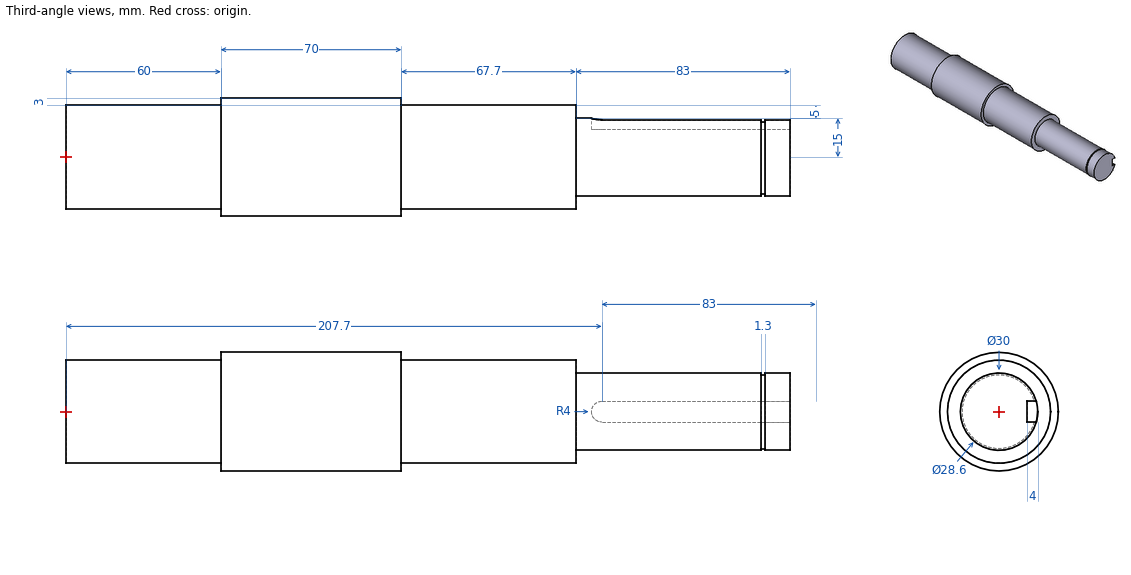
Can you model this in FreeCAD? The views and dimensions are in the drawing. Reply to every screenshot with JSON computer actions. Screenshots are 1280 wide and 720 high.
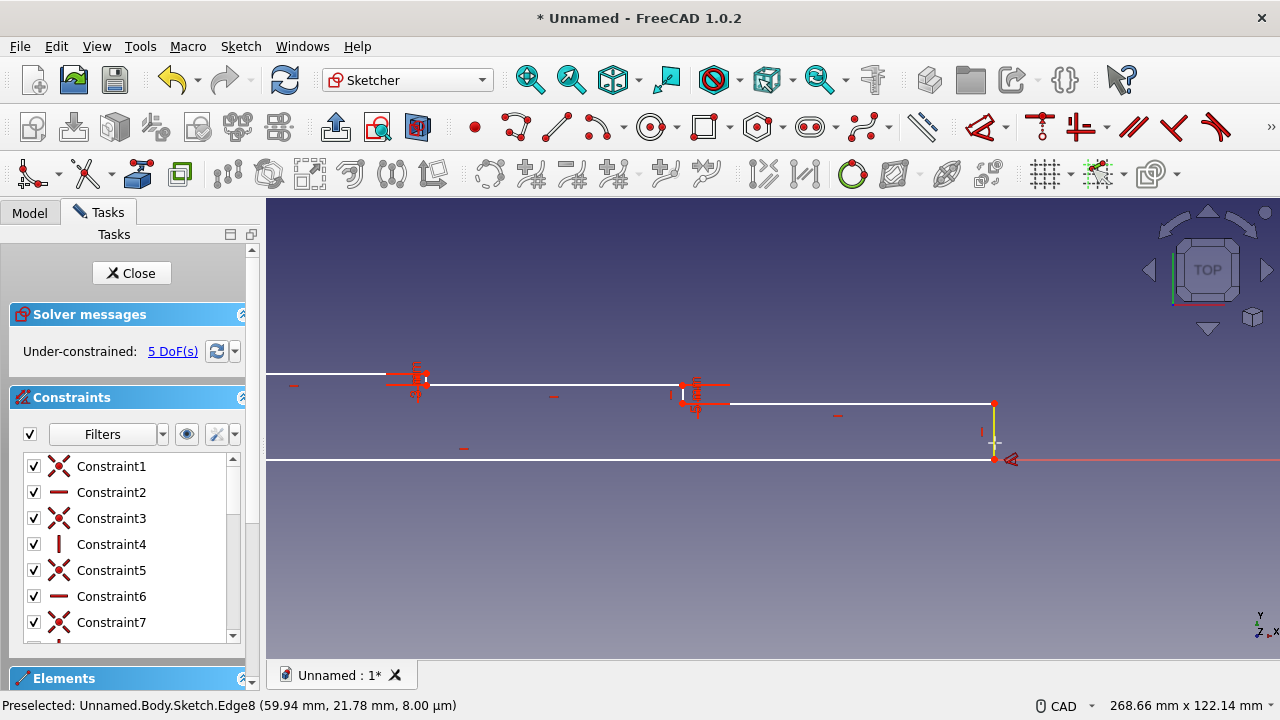
{"action": "left_click", "coordinate": [994, 443]}
{"action": "left_click", "coordinate": [1028, 432]}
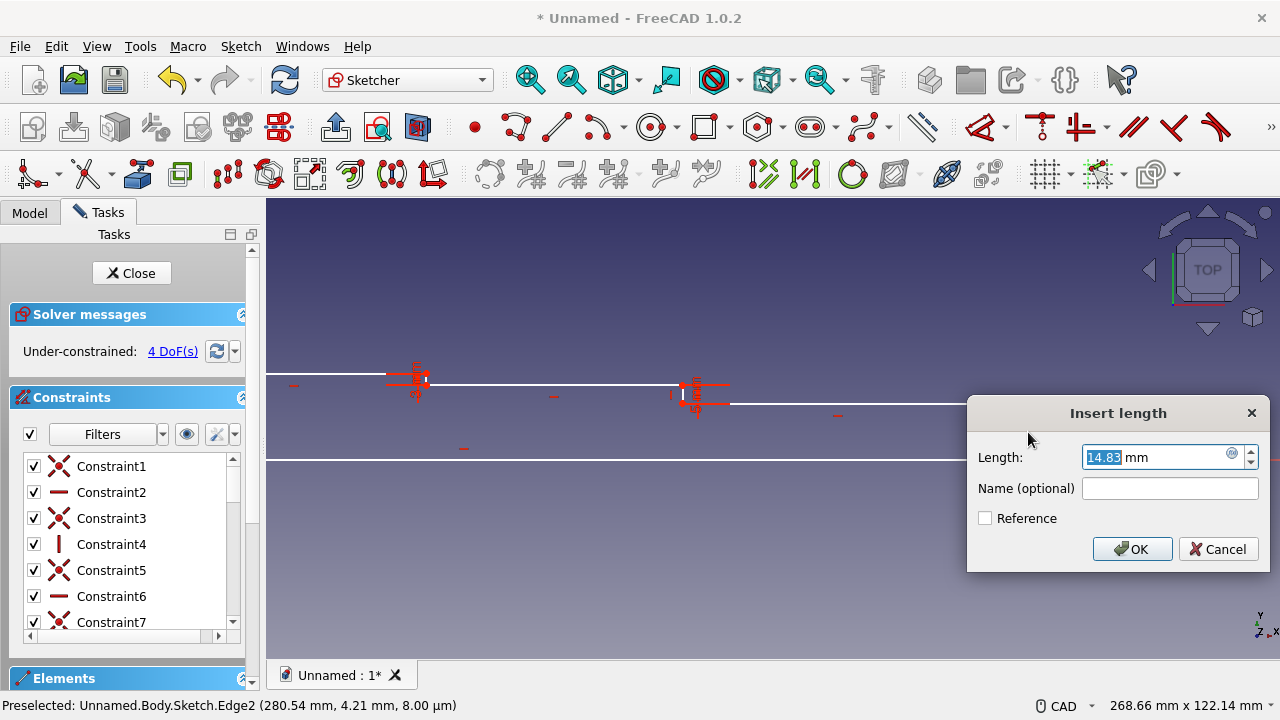
{"action": "type", "text": "15"}
{"action": "key", "text": "Return"}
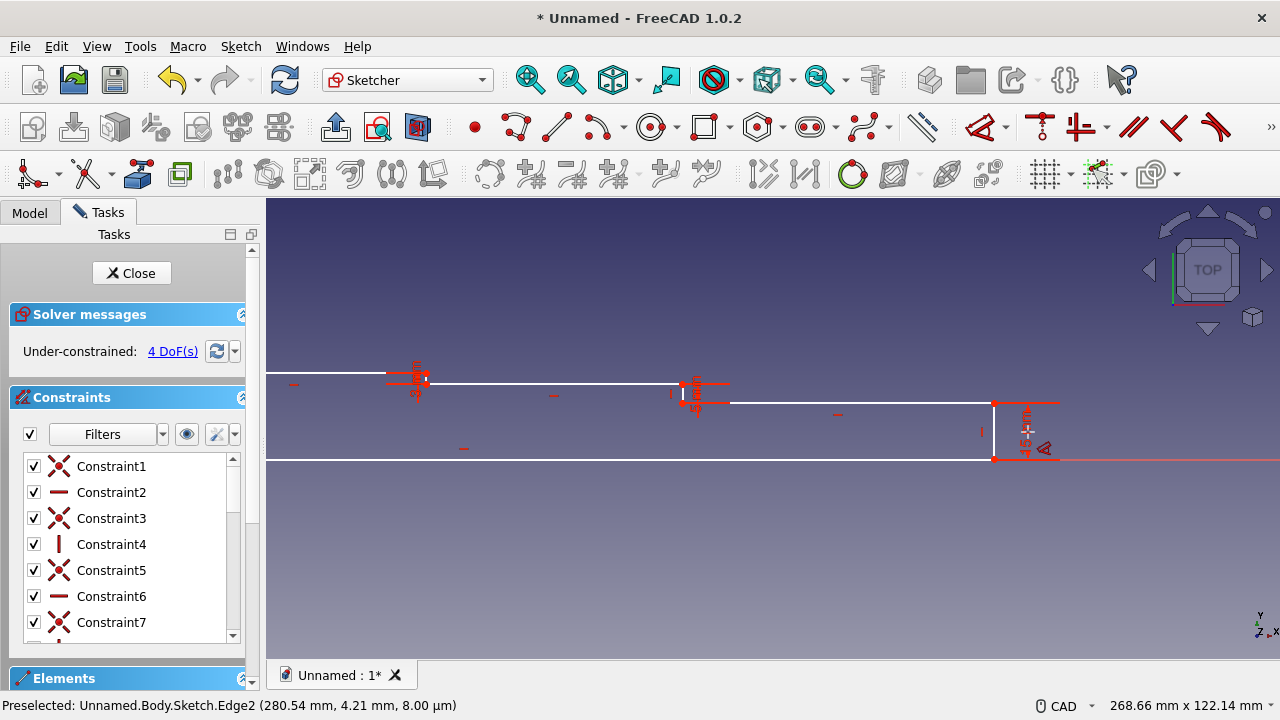
{"action": "left_click", "coordinate": [901, 403]}
{"action": "left_click", "coordinate": [839, 369]}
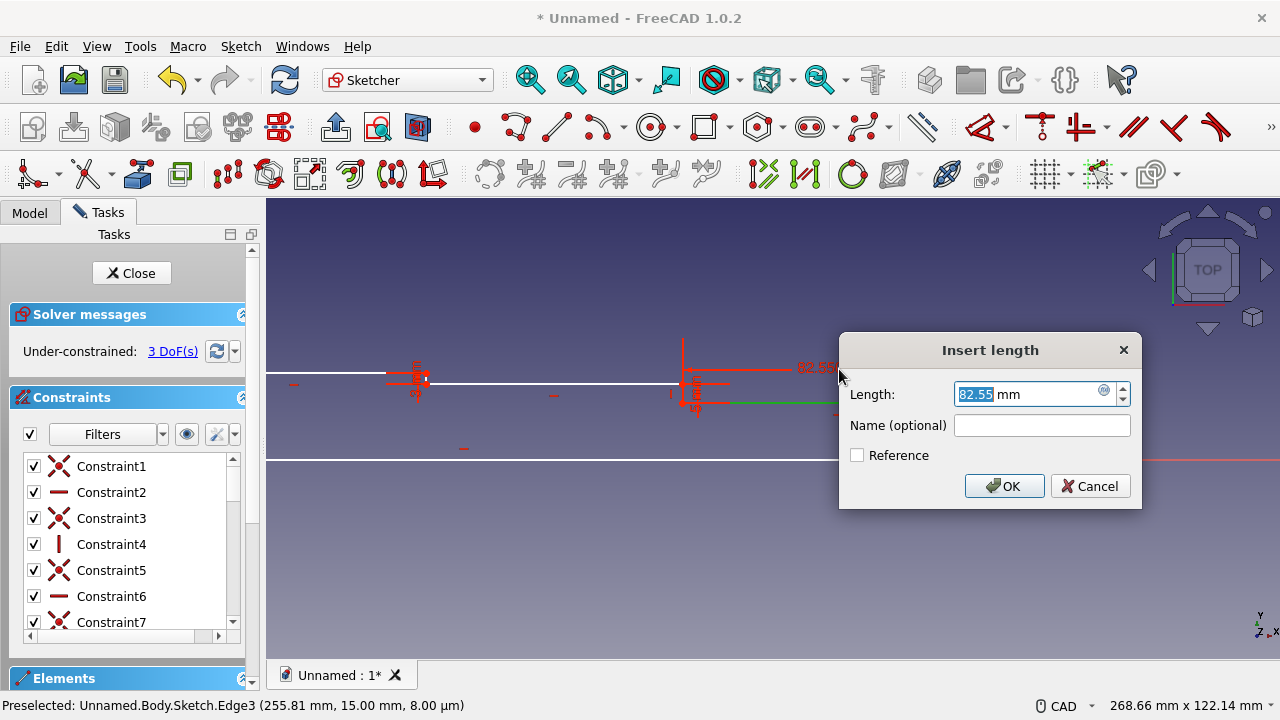
{"action": "type", "text": "83"}
{"action": "key", "text": "Return"}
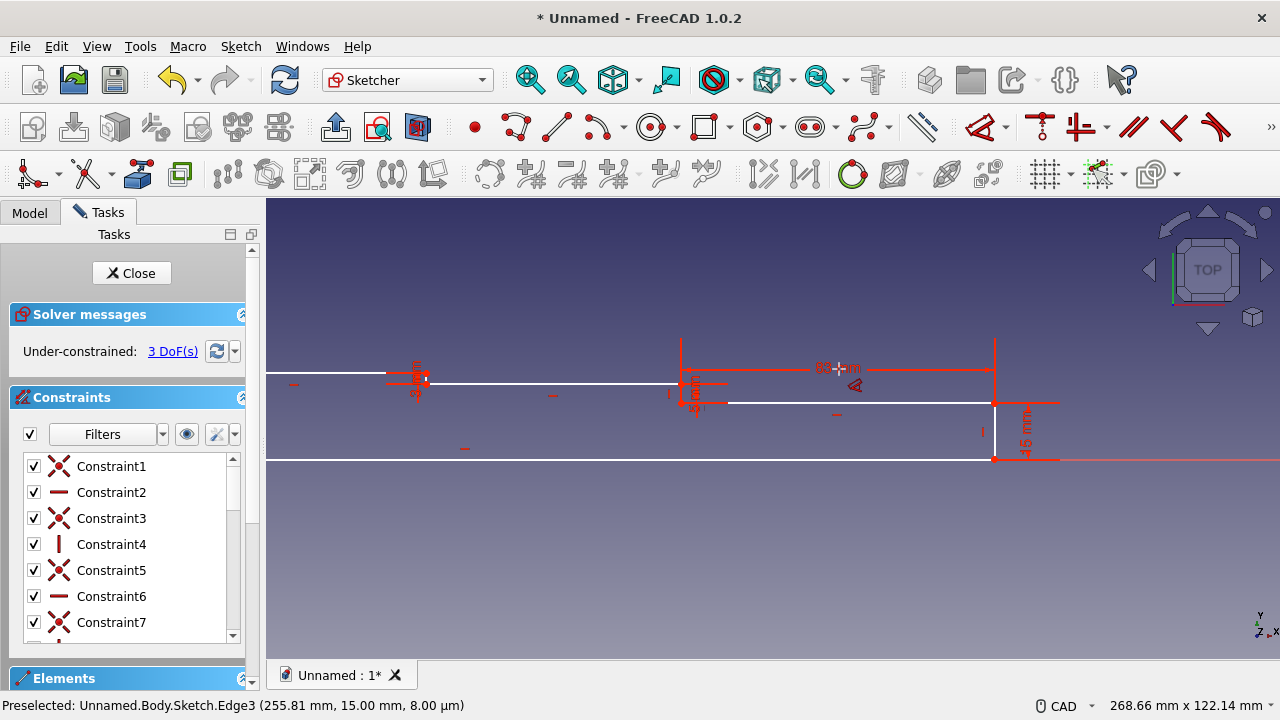
{"action": "left_click", "coordinate": [347, 373]}
{"action": "left_click", "coordinate": [360, 339]}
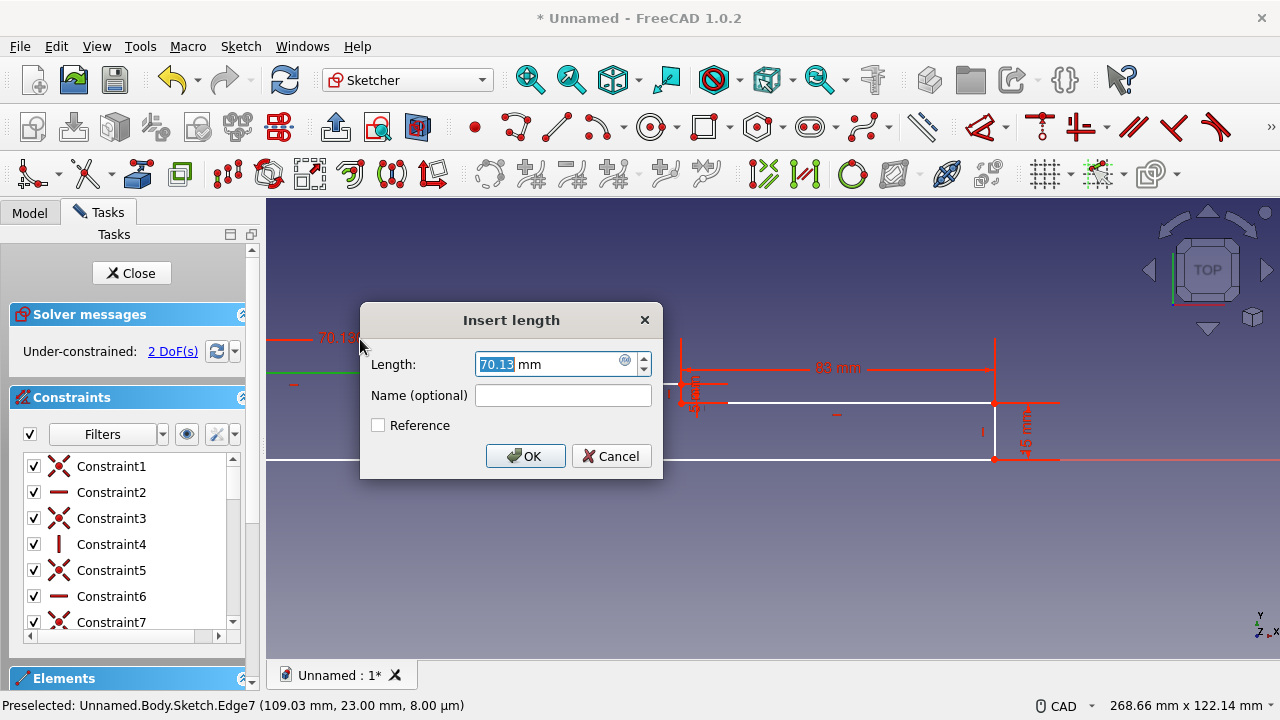
{"action": "type", "text": "70"}
{"action": "key", "text": "Return"}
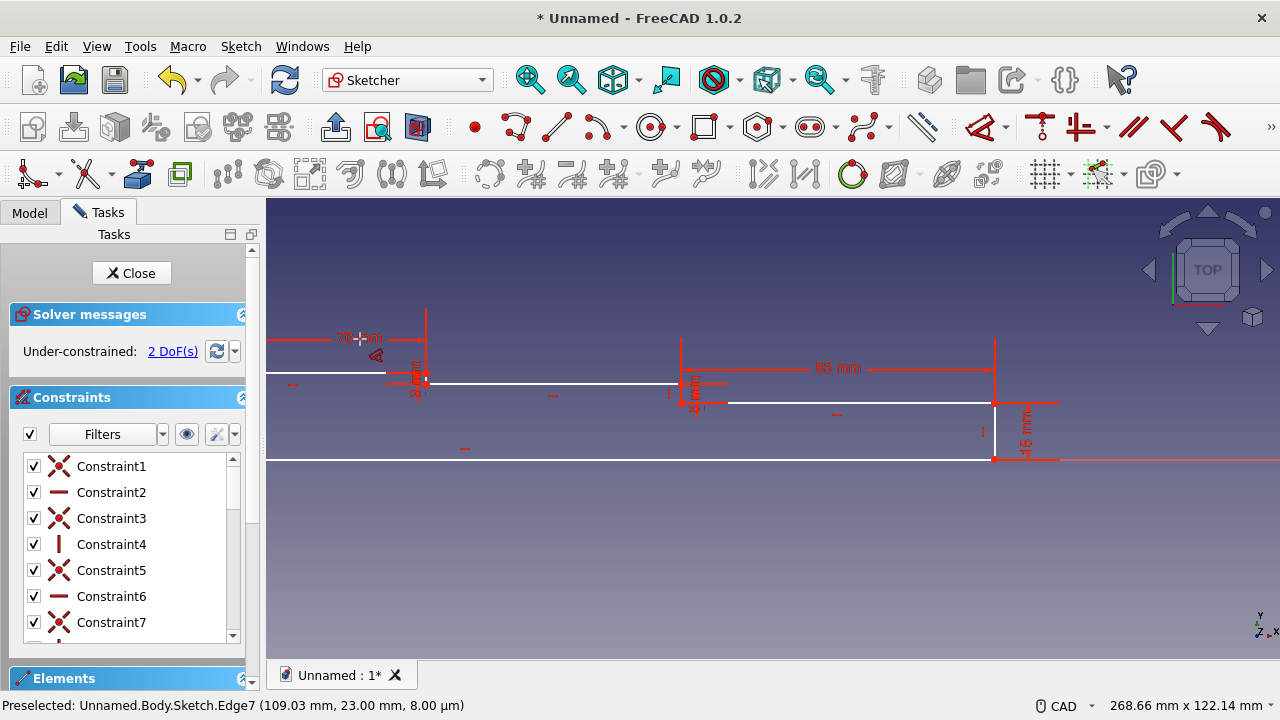
{"action": "scroll", "coordinate": [996, 443], "scroll_direction": "down", "scroll_amount": 3}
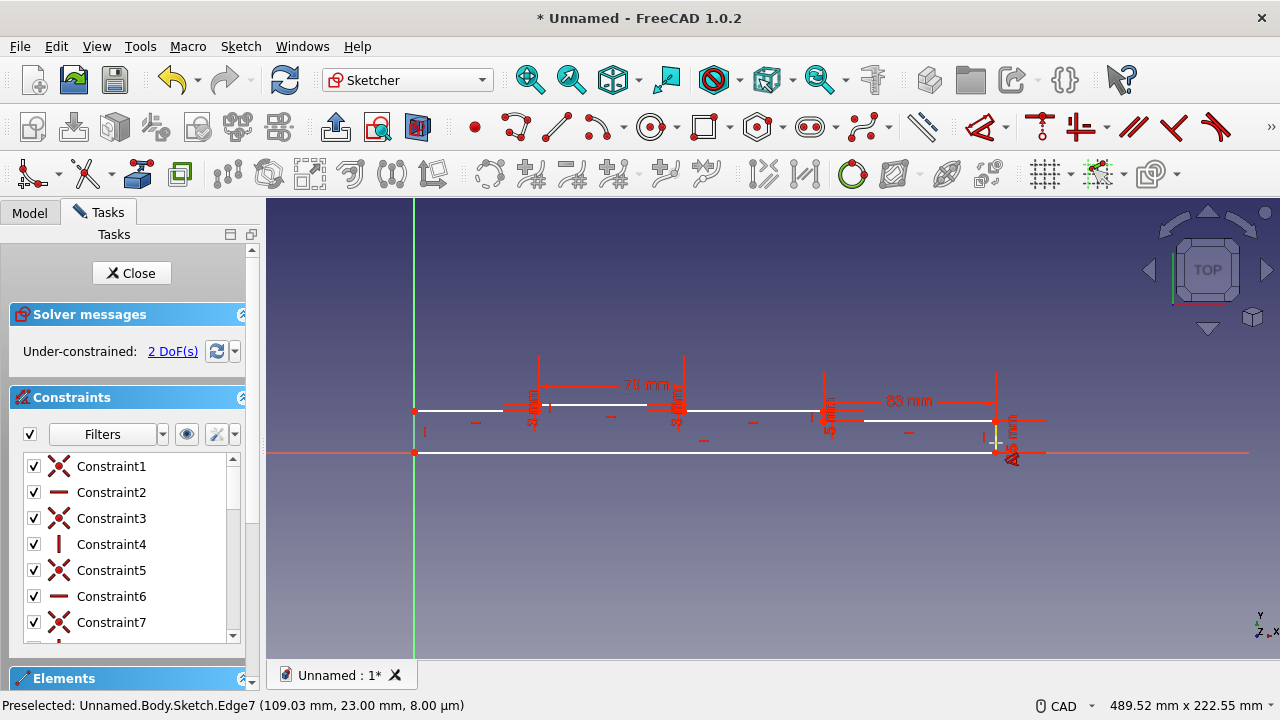
{"action": "left_click", "coordinate": [501, 411]}
{"action": "left_click", "coordinate": [476, 377]}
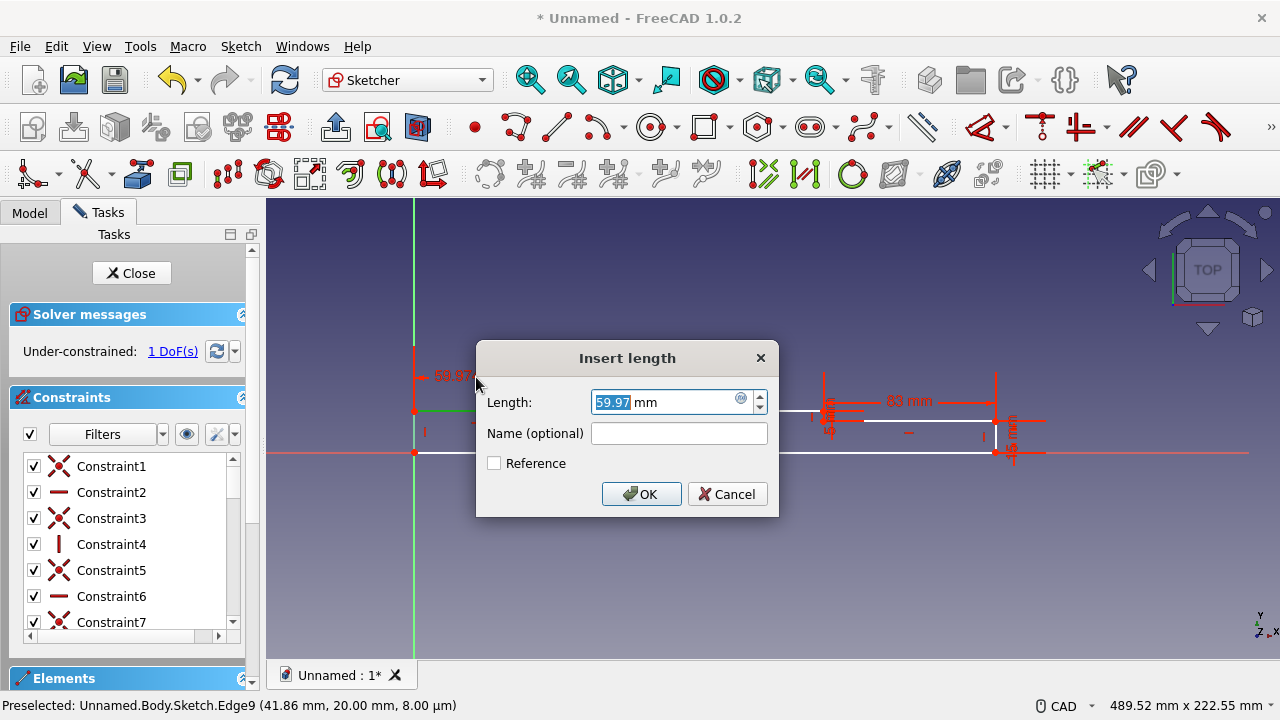
{"action": "type", "text": "60"}
{"action": "key", "text": "Return"}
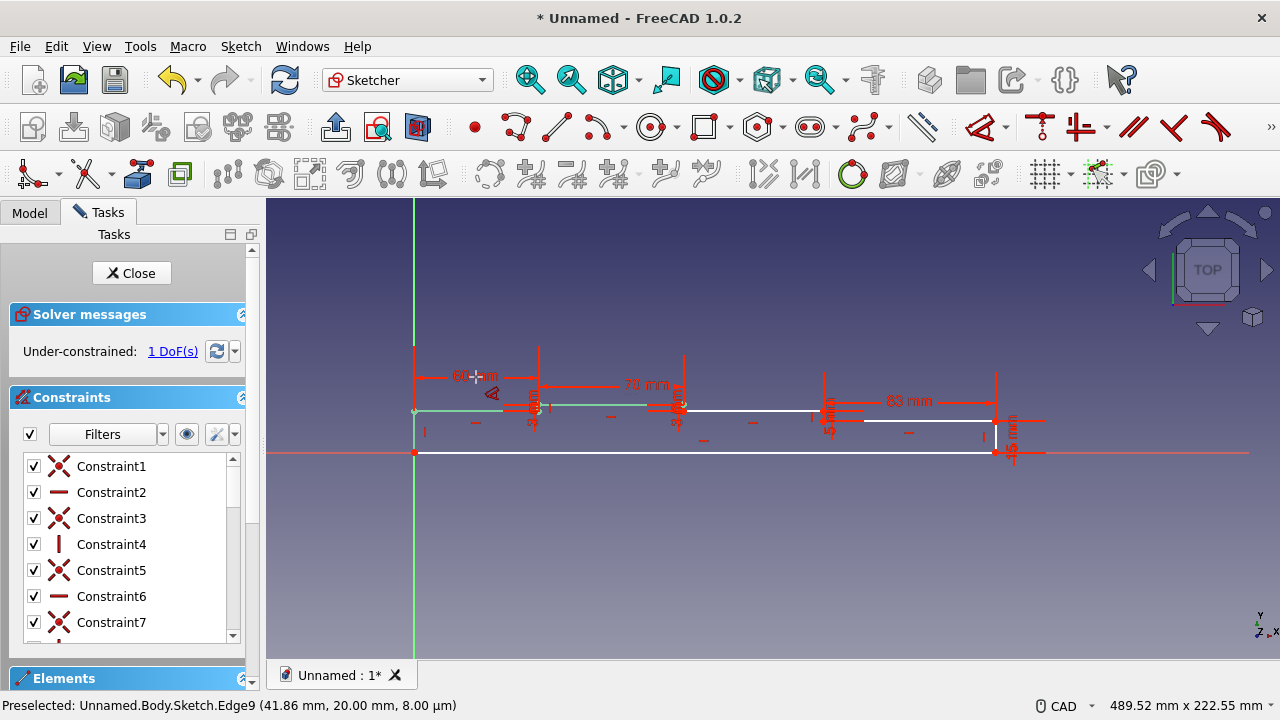
{"action": "left_click", "coordinate": [782, 411]}
{"action": "left_click", "coordinate": [754, 377]}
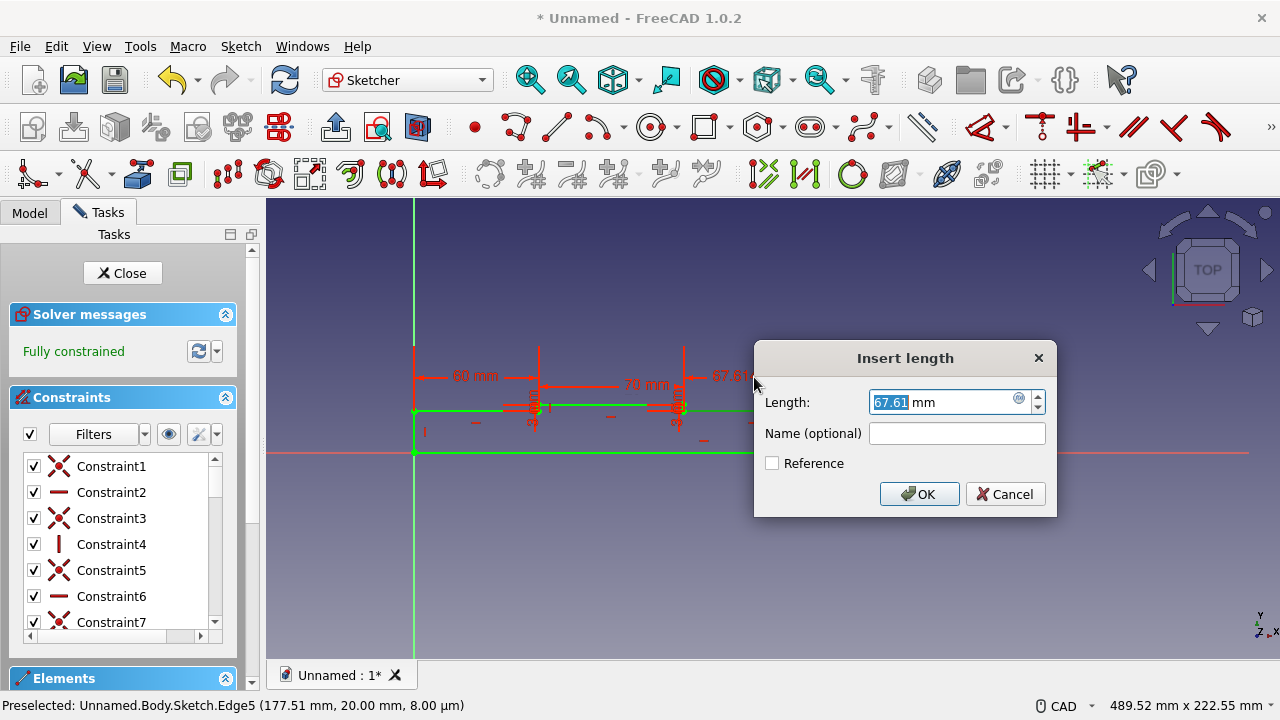
{"action": "type", "text": "67.7"}
{"action": "key", "text": "Return"}
{"action": "key", "text": "Escape"}